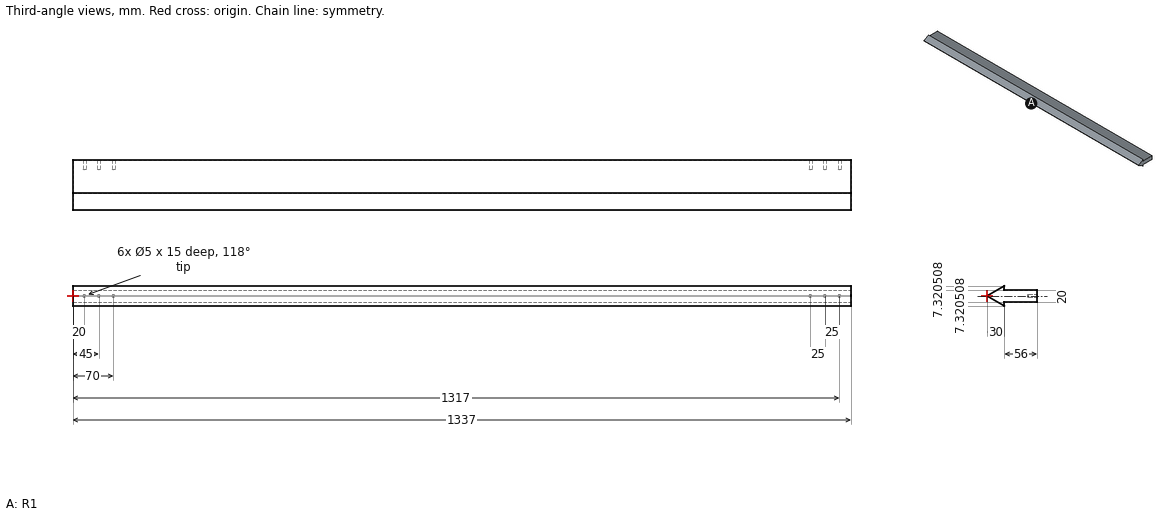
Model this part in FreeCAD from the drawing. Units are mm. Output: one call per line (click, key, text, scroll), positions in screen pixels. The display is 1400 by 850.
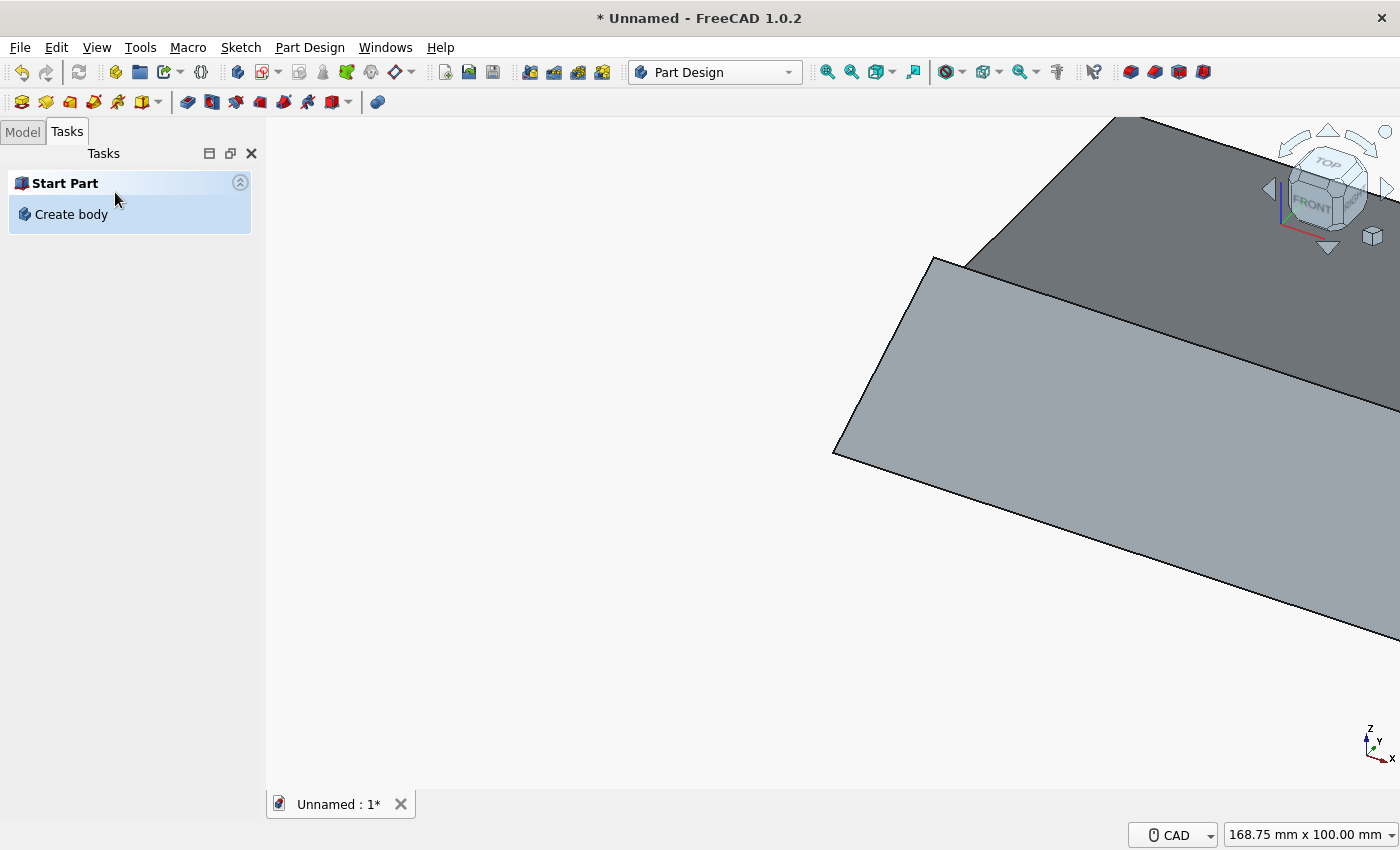
click(828, 72)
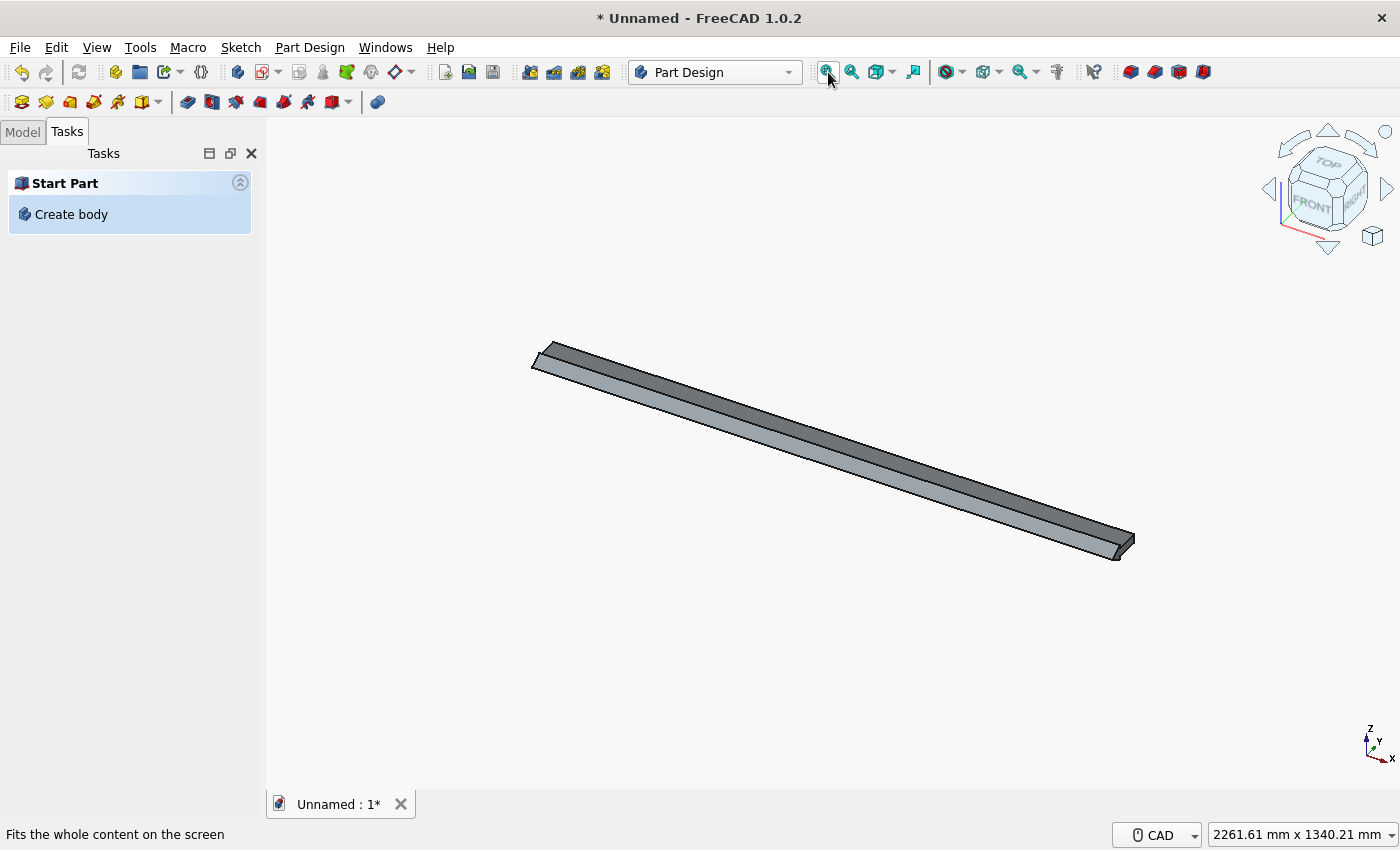
click(822, 463)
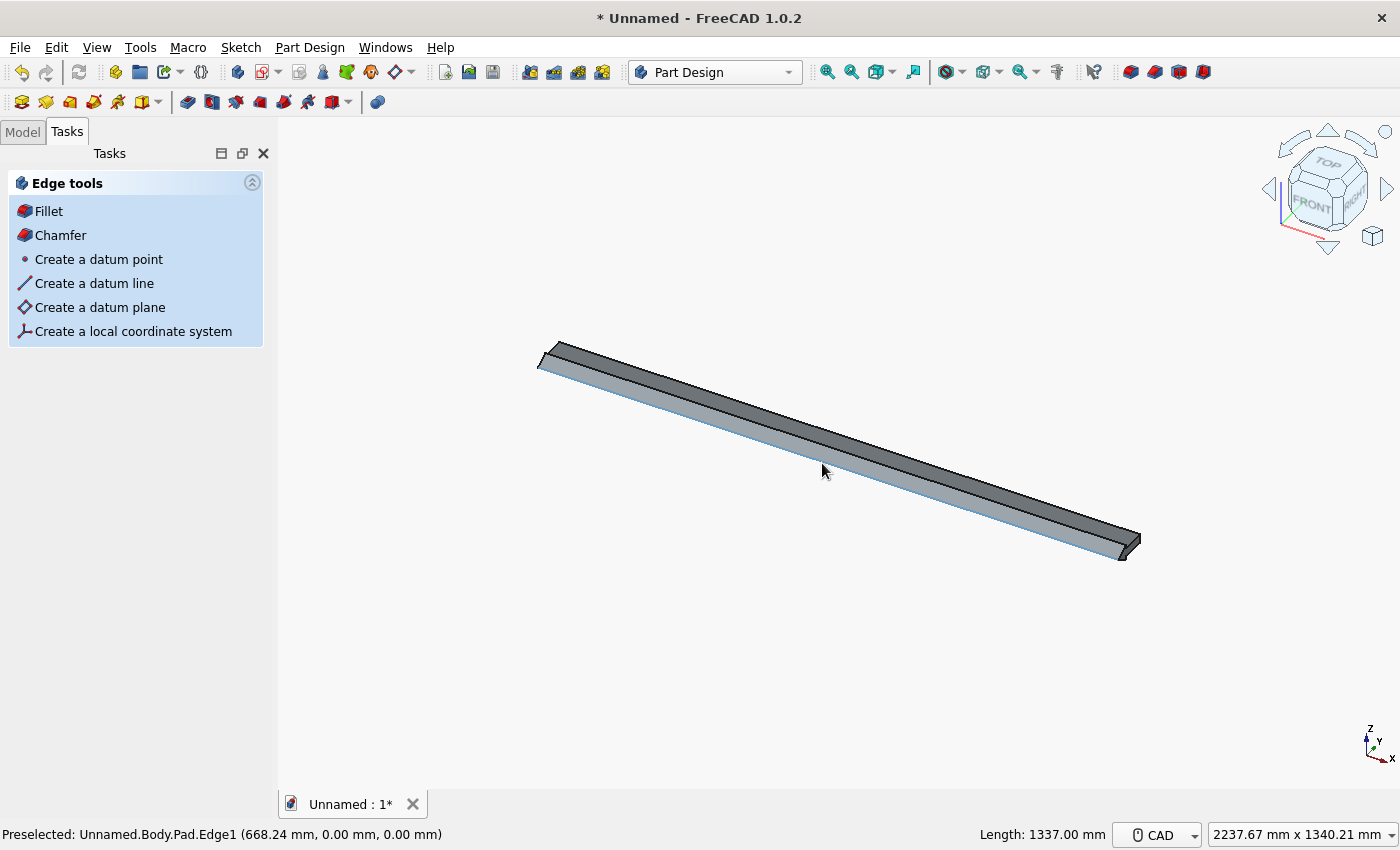
click(1132, 72)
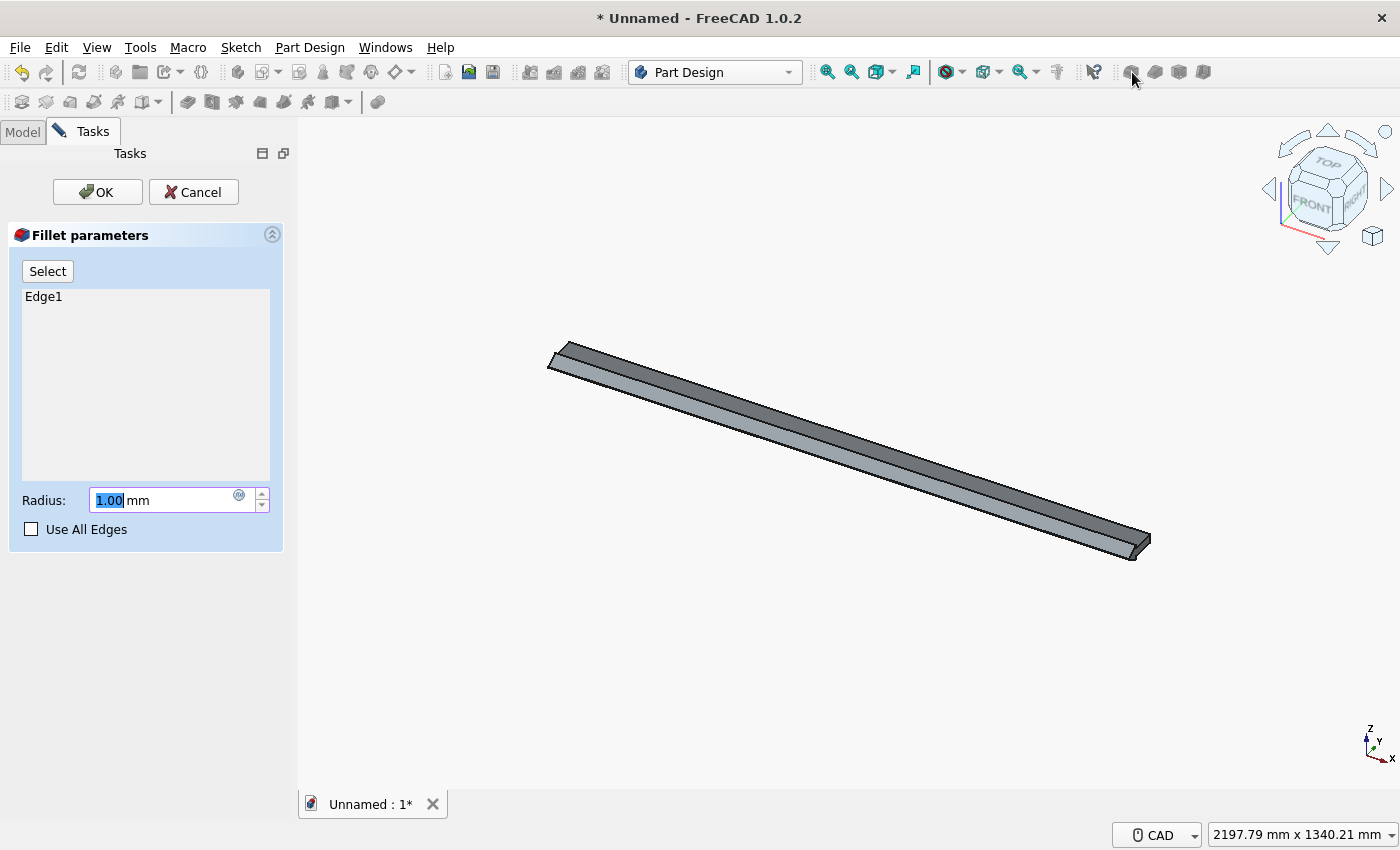
text(1)
key(Tab)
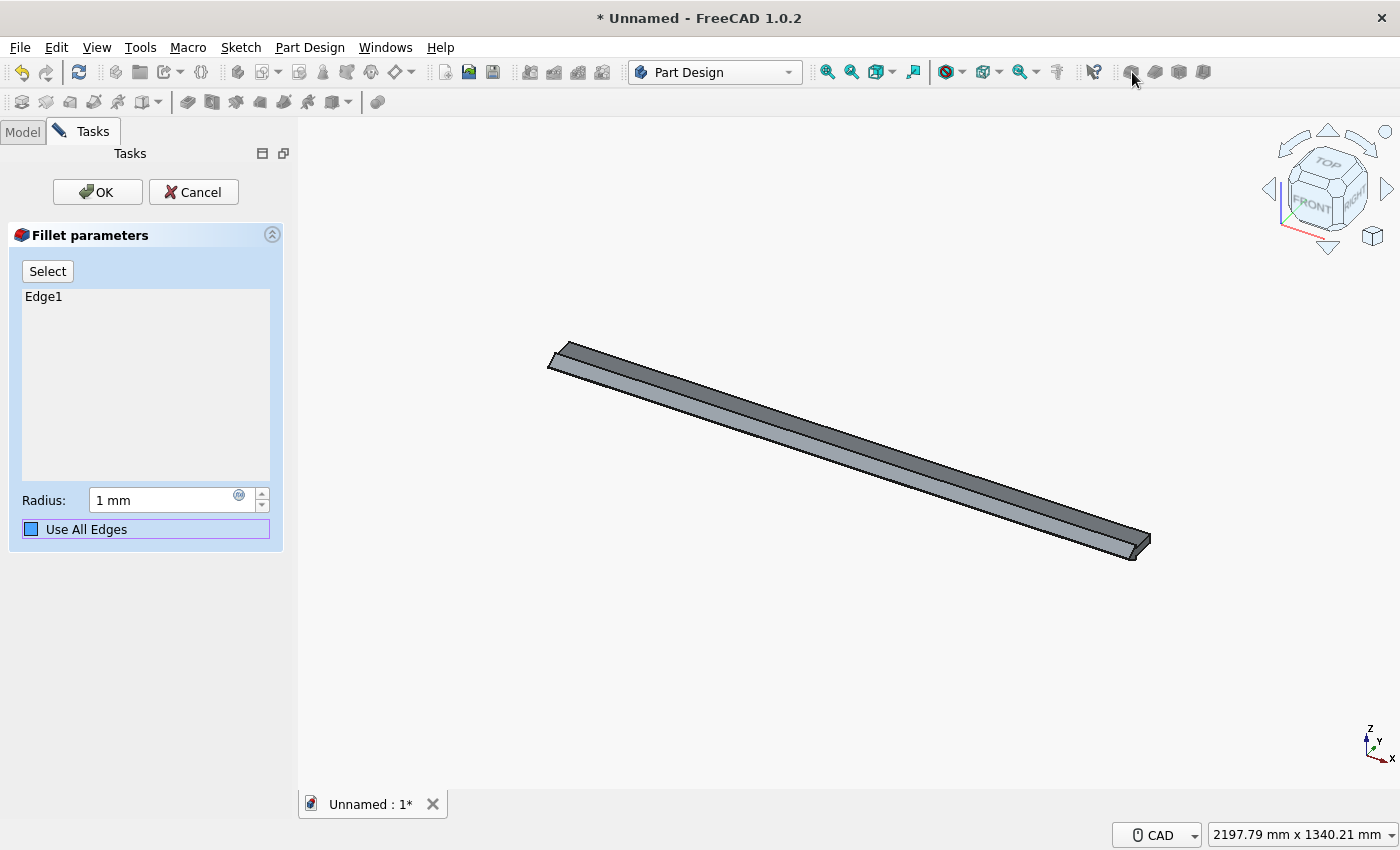
click(98, 192)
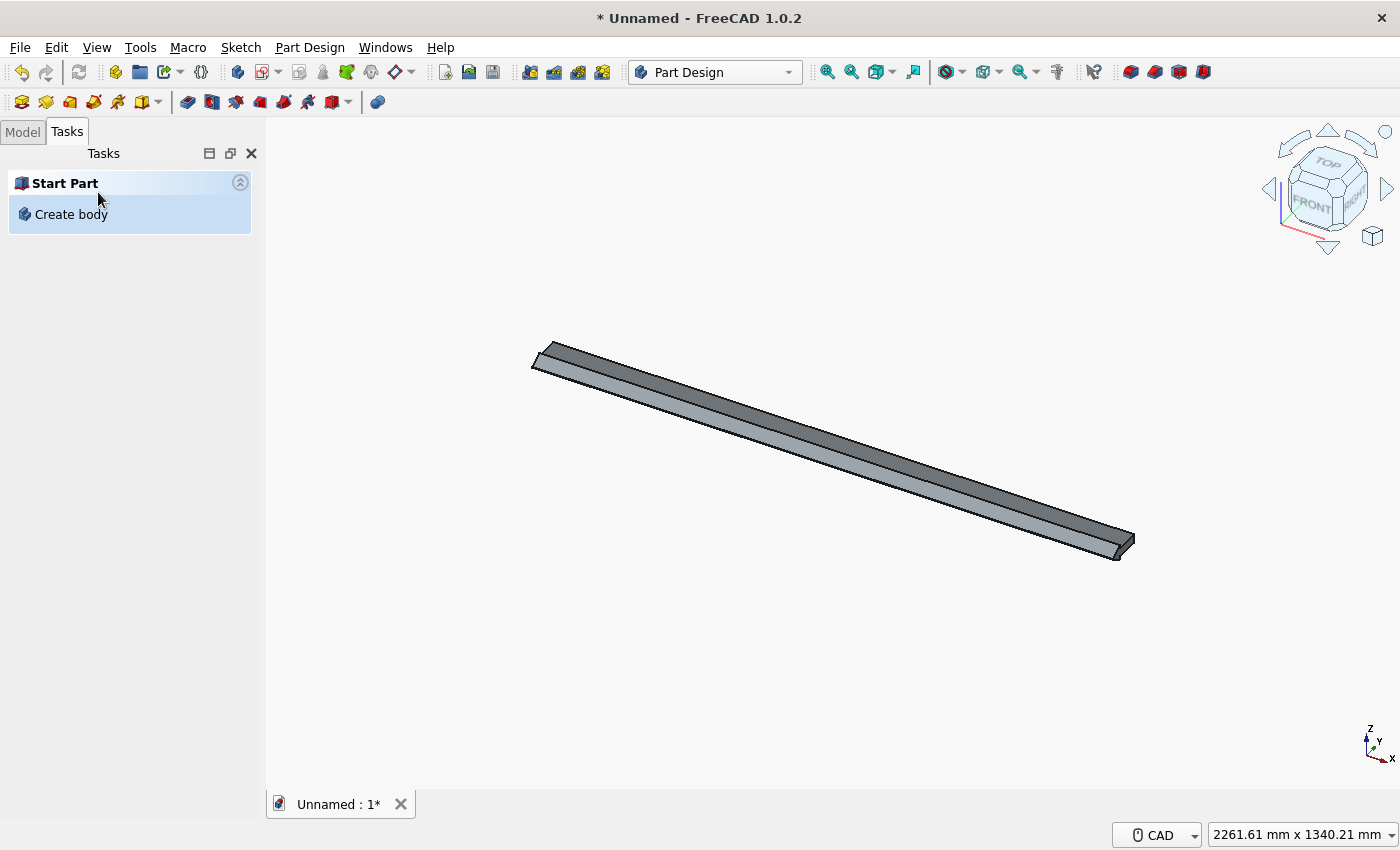
key(4)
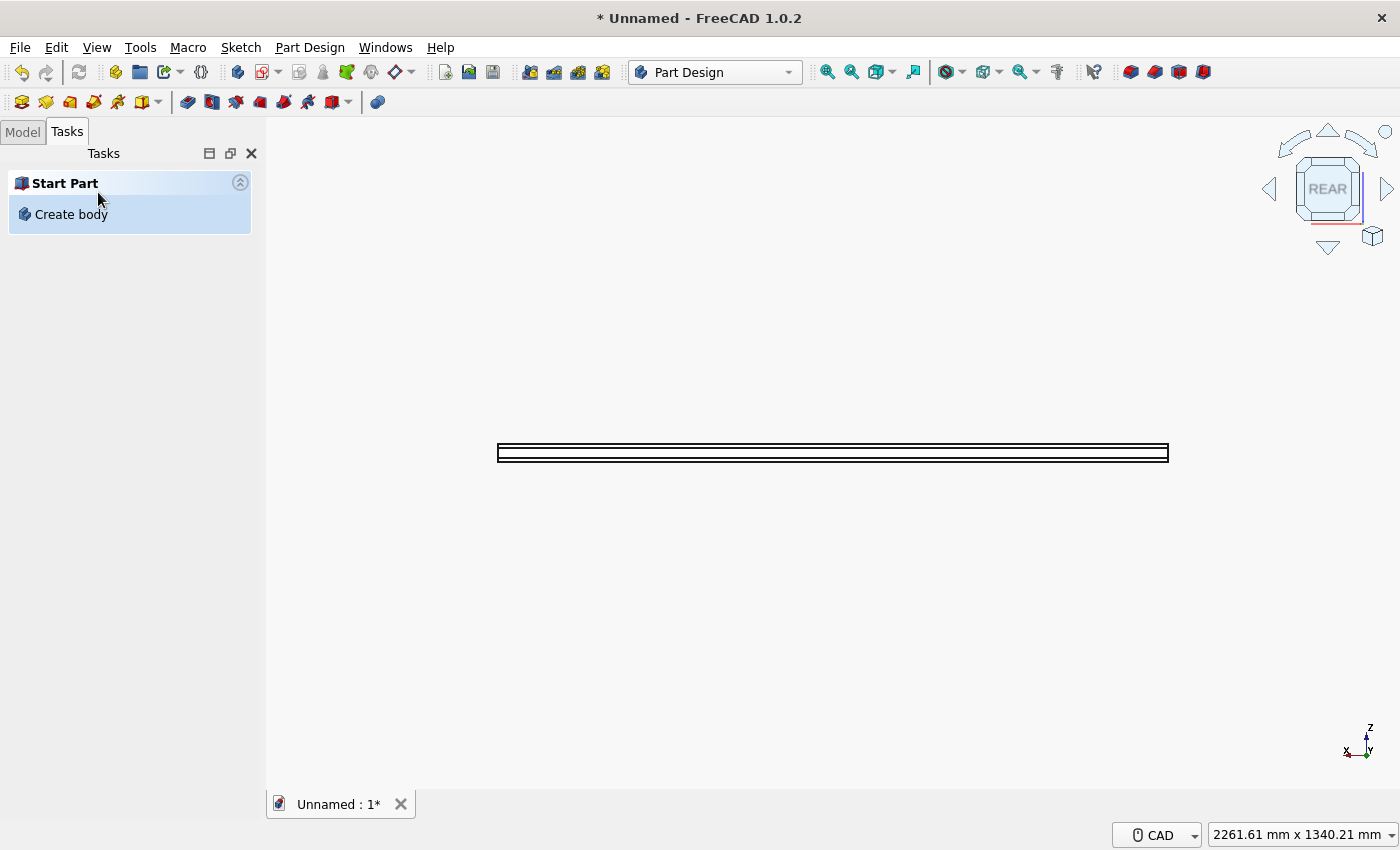
scroll(833, 452, up, 5)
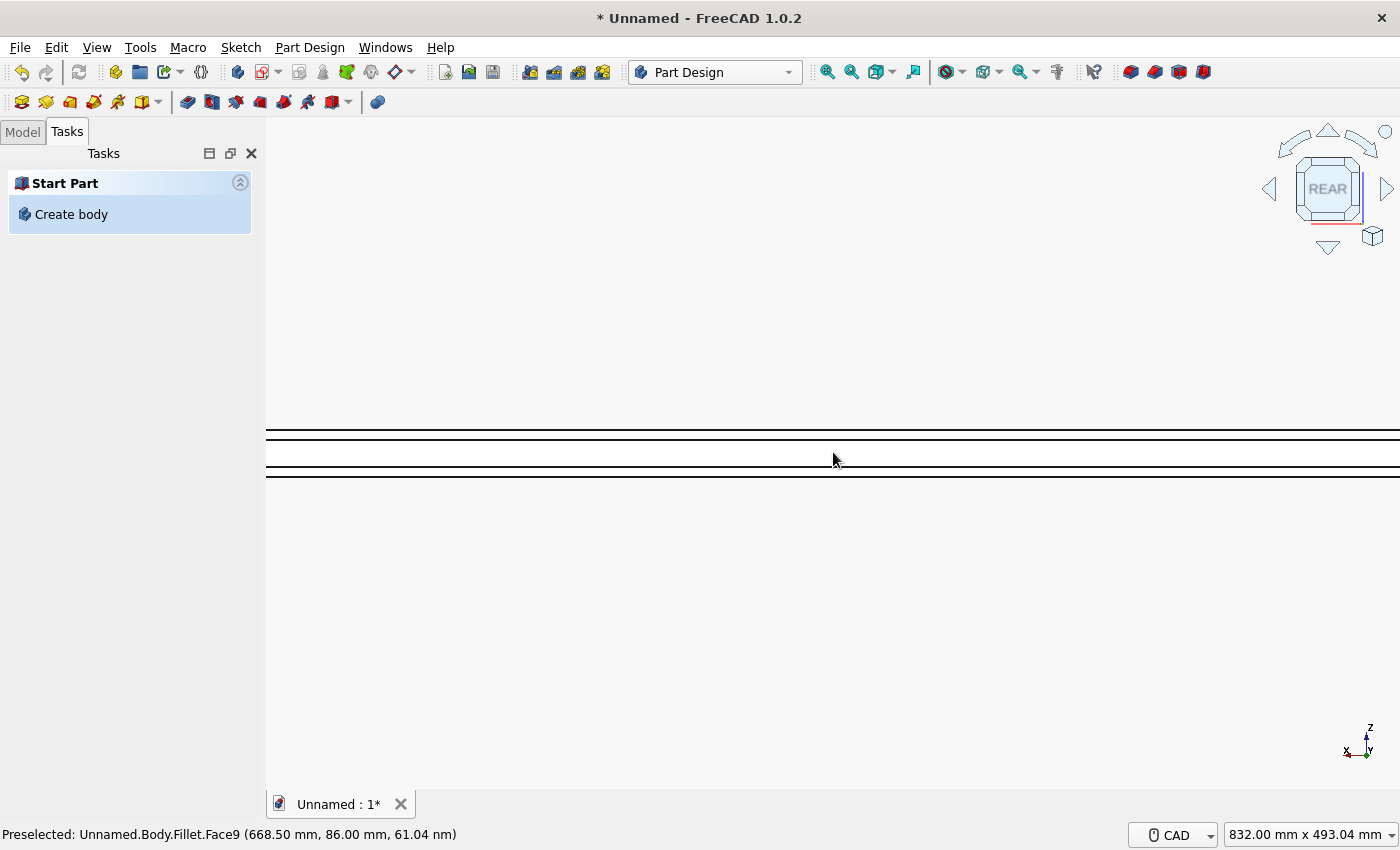
click(832, 453)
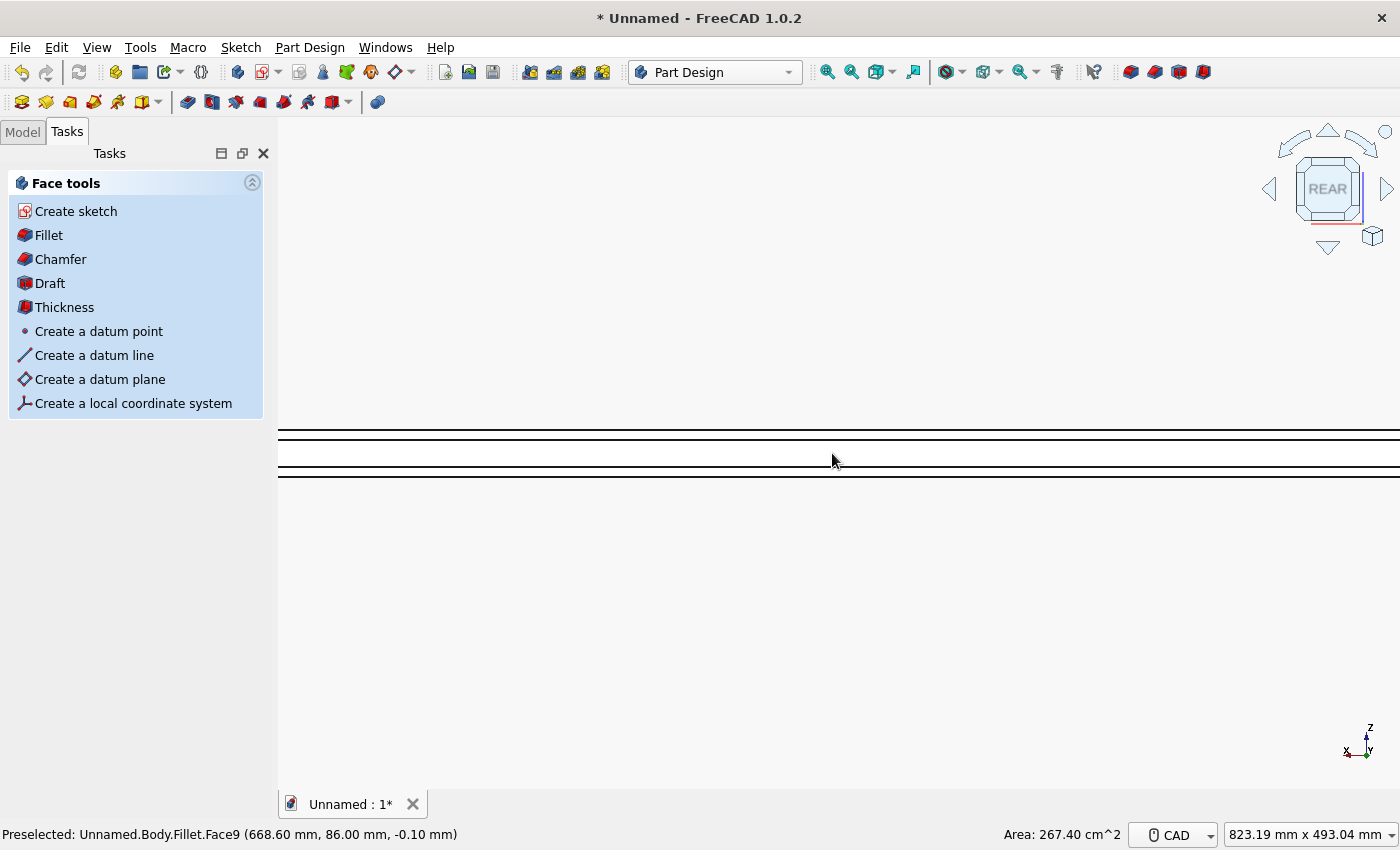
click(262, 72)